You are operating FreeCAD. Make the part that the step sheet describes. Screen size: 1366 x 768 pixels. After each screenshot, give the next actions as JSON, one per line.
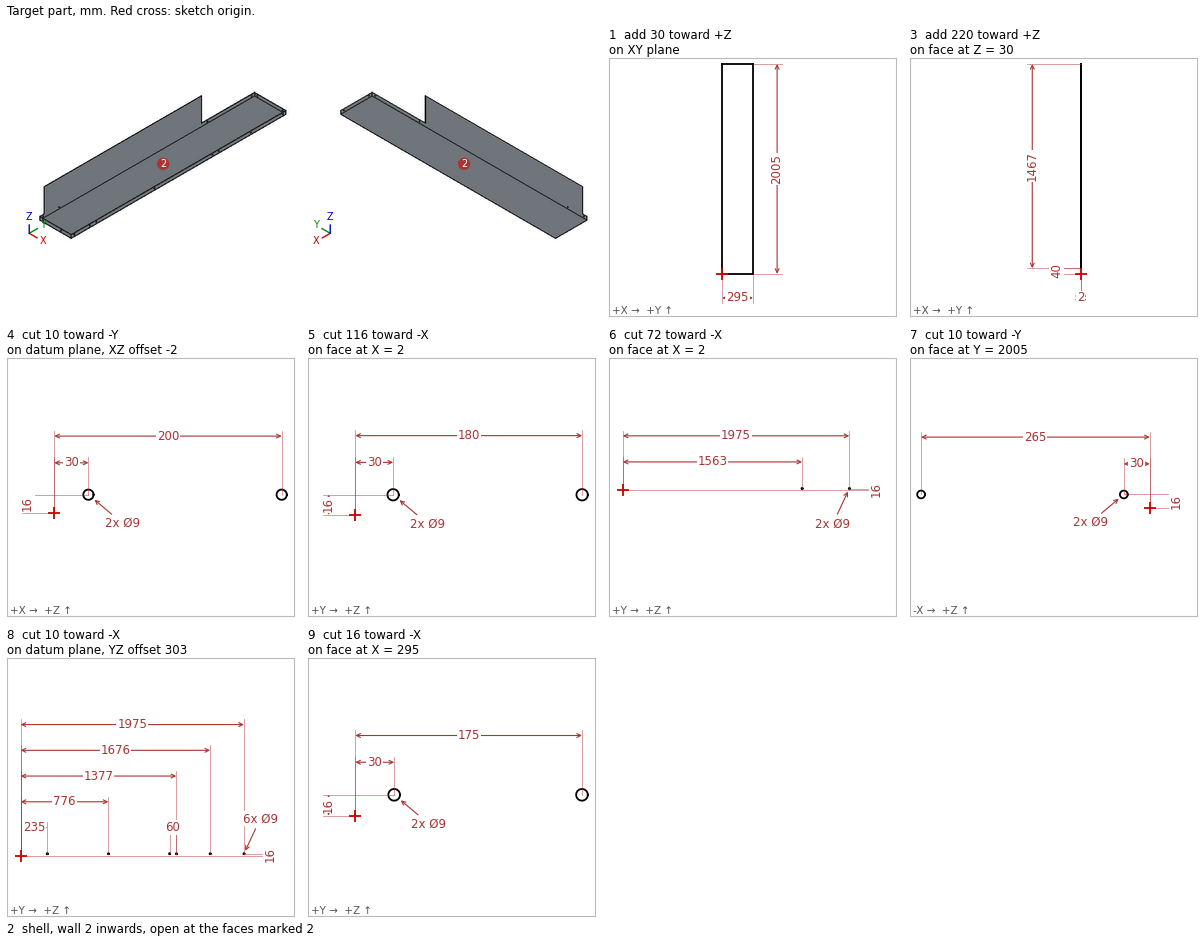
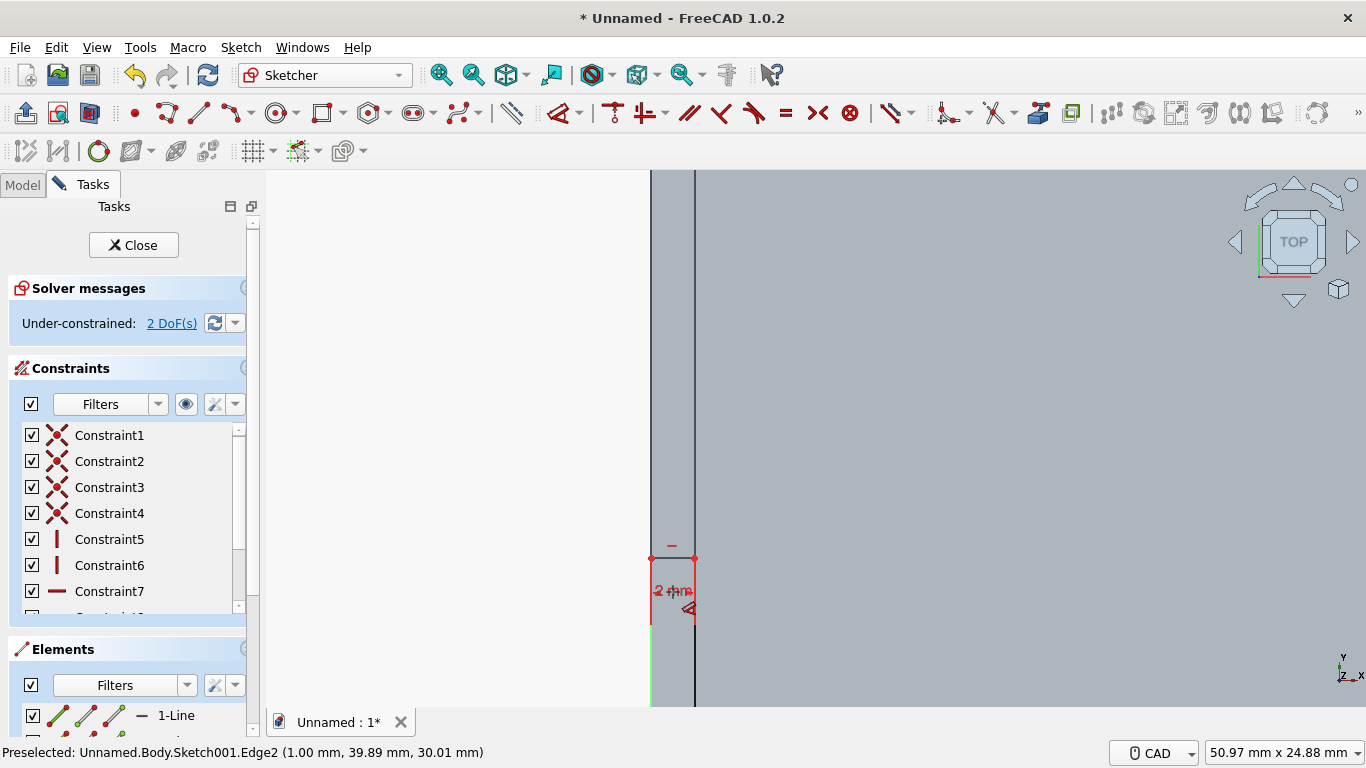
{"action": "scroll", "coordinate": [748, 438], "scroll_direction": "down", "scroll_amount": 15}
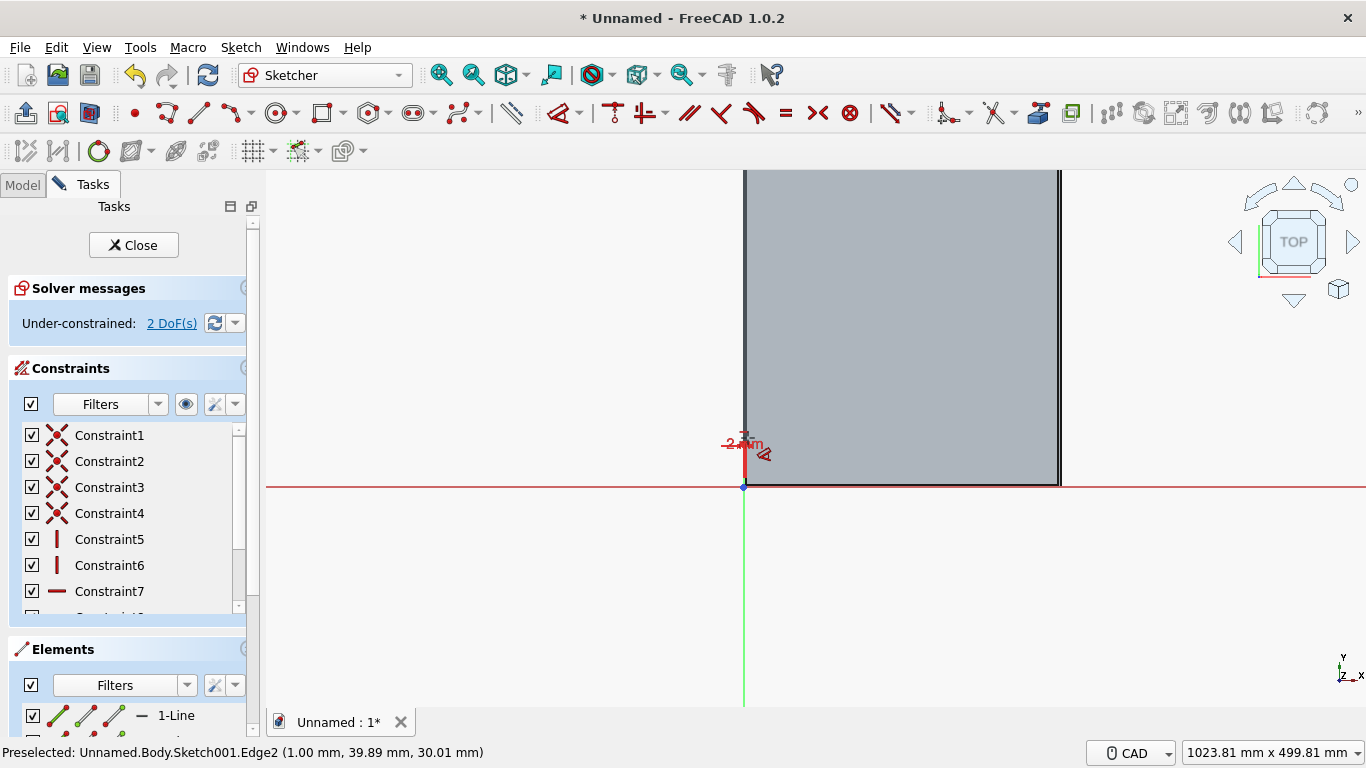
{"action": "scroll", "coordinate": [748, 631], "scroll_direction": "down", "scroll_amount": 8}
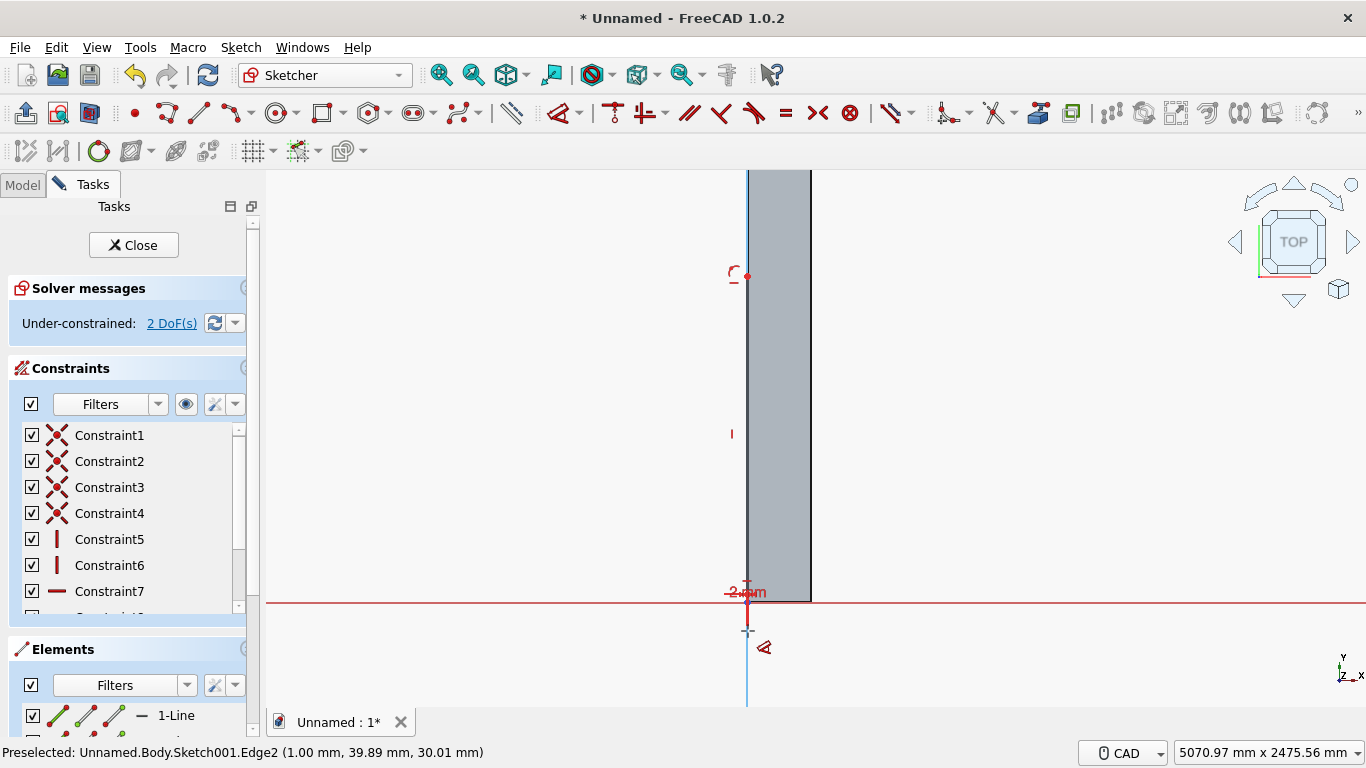
{"action": "scroll", "coordinate": [747, 594], "scroll_direction": "up", "scroll_amount": 14}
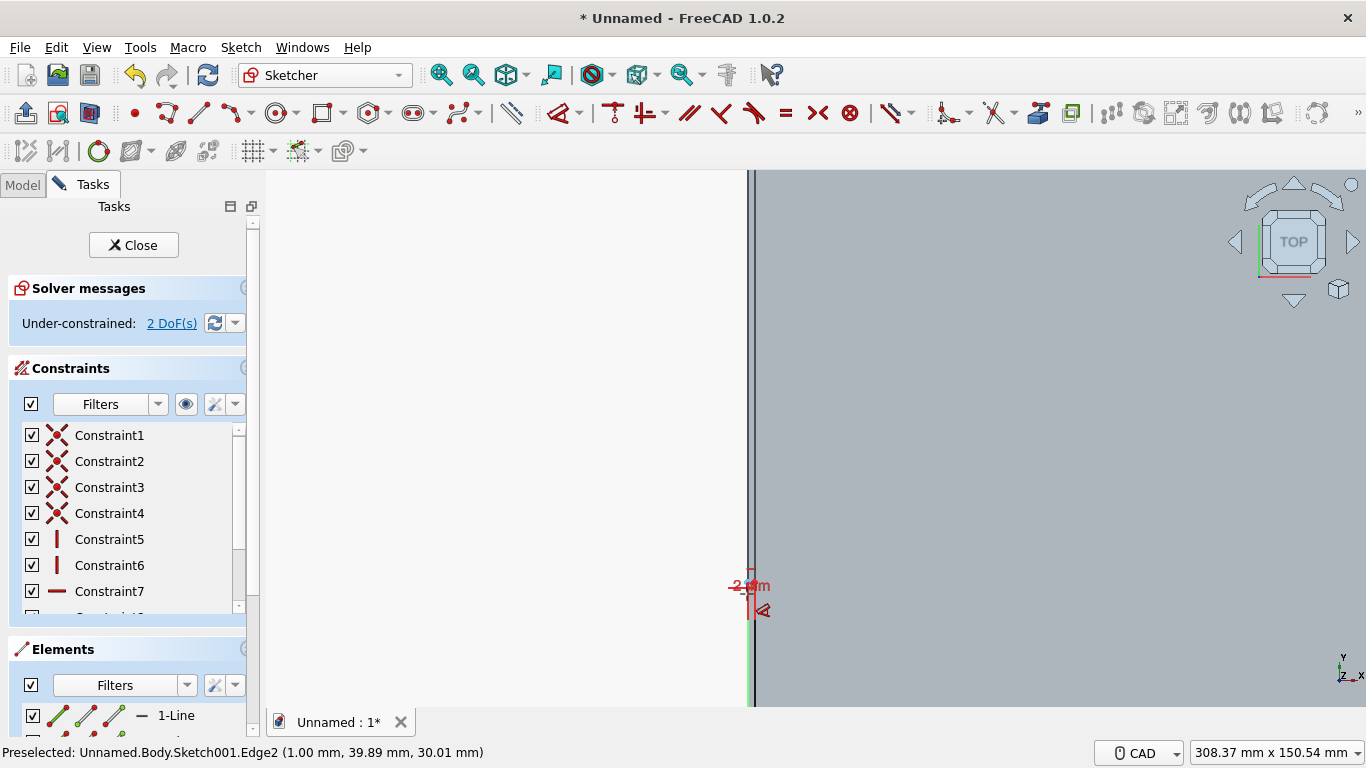
{"action": "left_click", "coordinate": [748, 582]}
{"action": "left_click", "coordinate": [714, 631]}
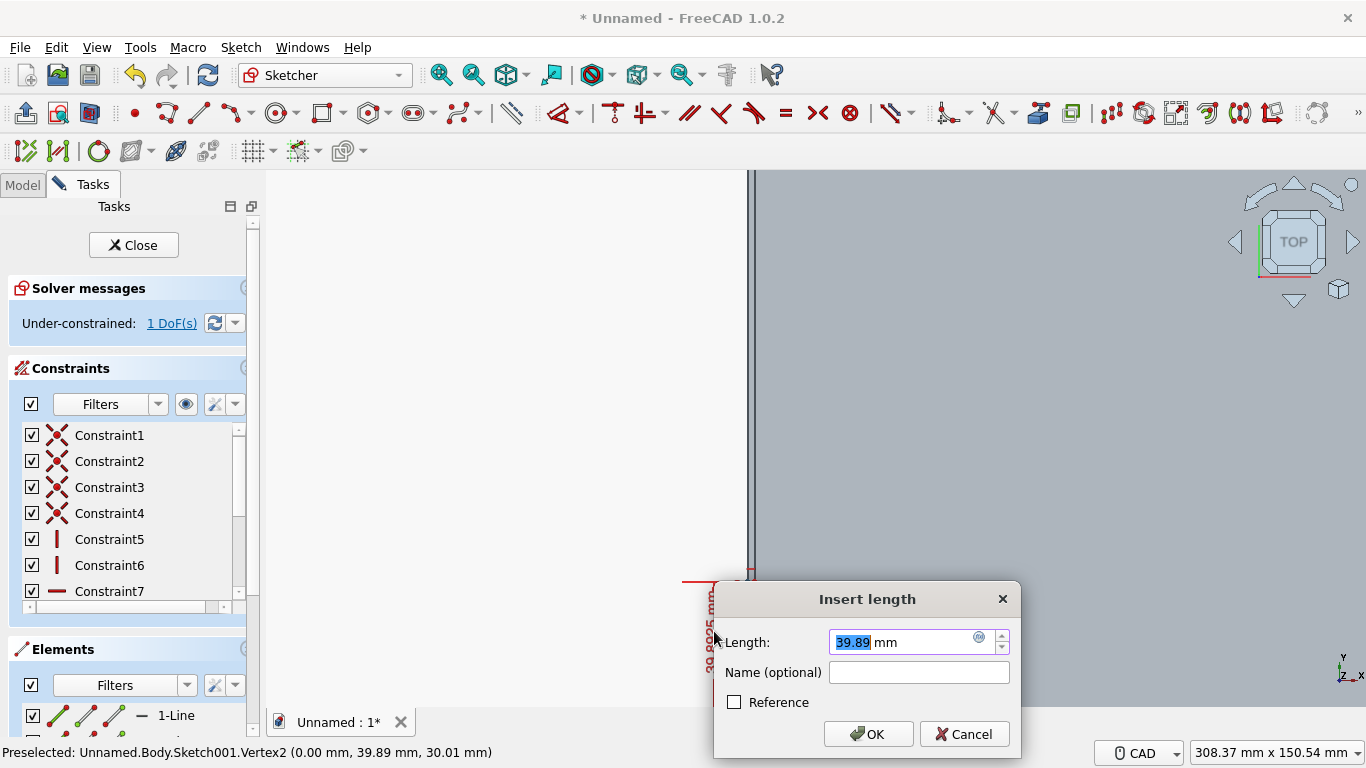
{"action": "type", "text": "40"}
{"action": "key", "text": "Return"}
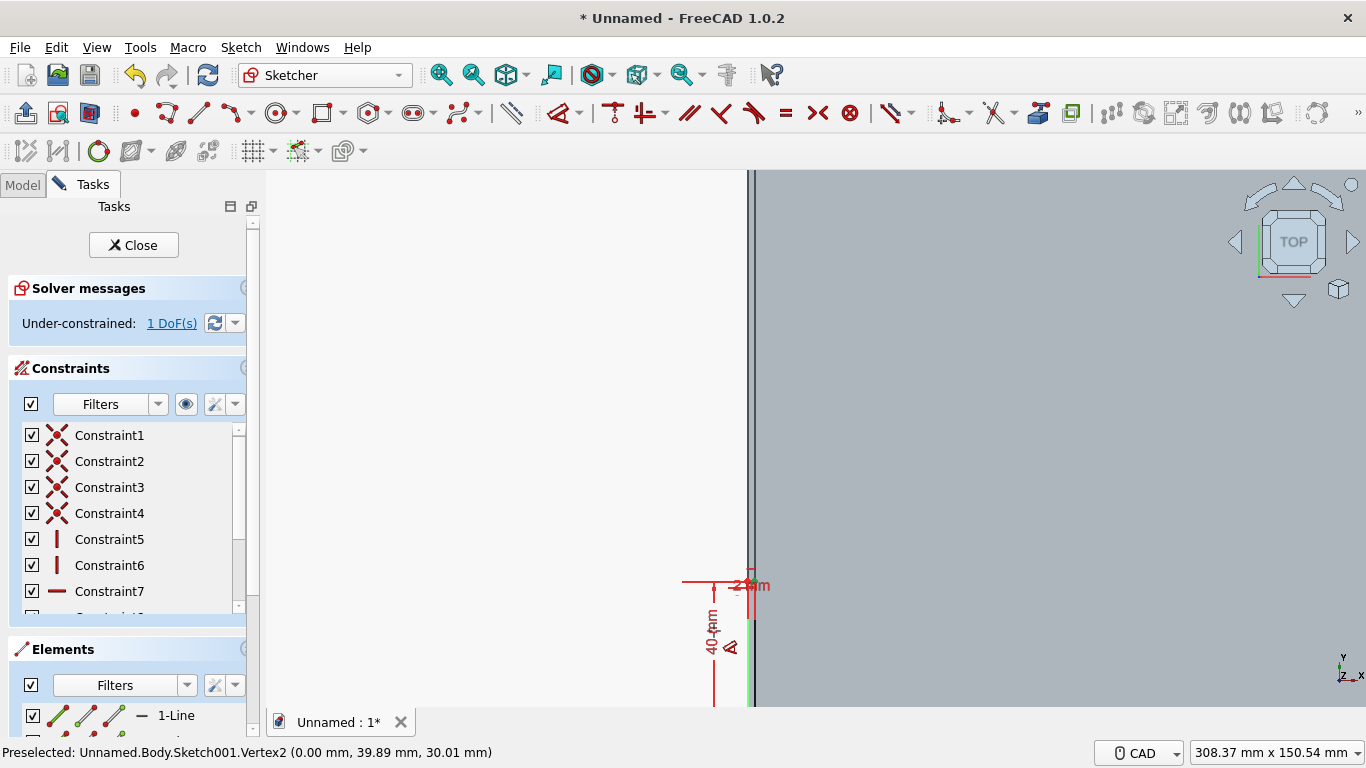
{"action": "scroll", "coordinate": [747, 594], "scroll_direction": "down", "scroll_amount": 14}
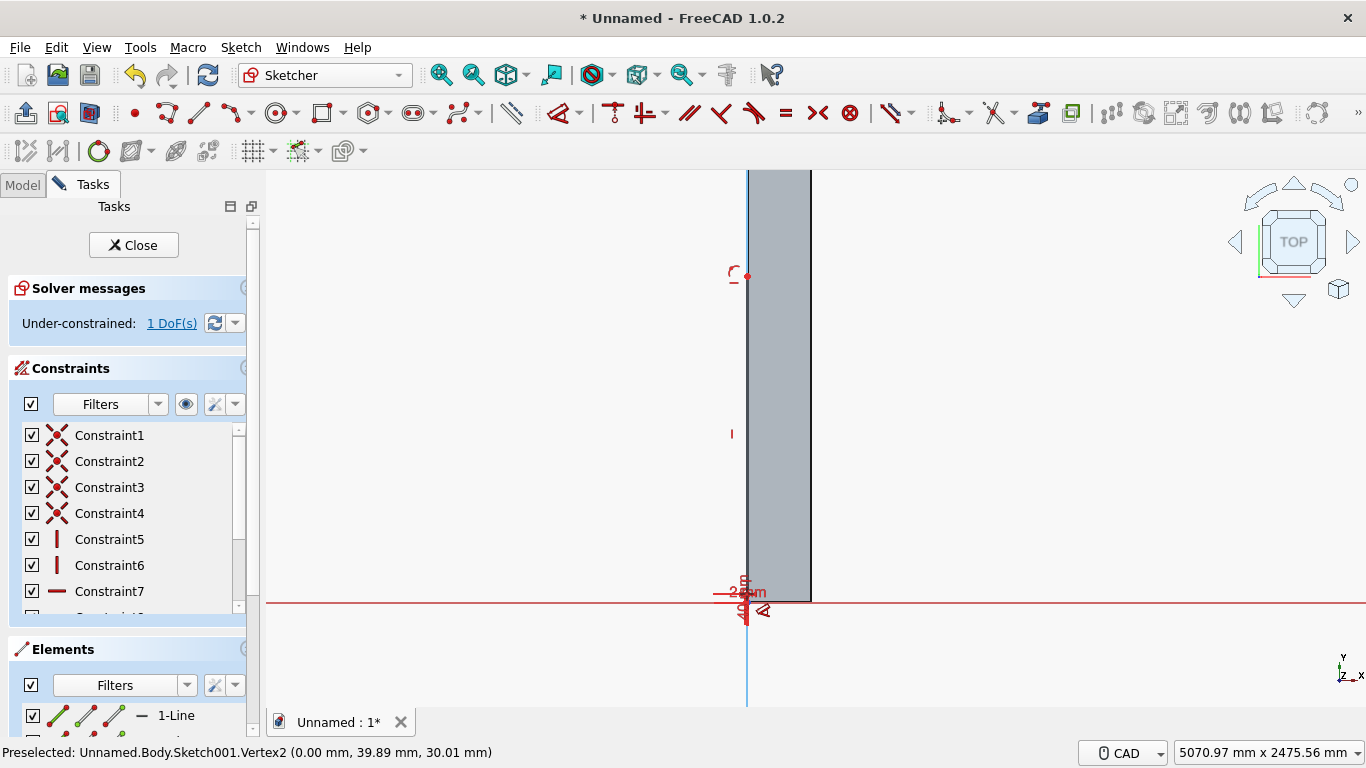
{"action": "scroll", "coordinate": [747, 372], "scroll_direction": "up", "scroll_amount": 14}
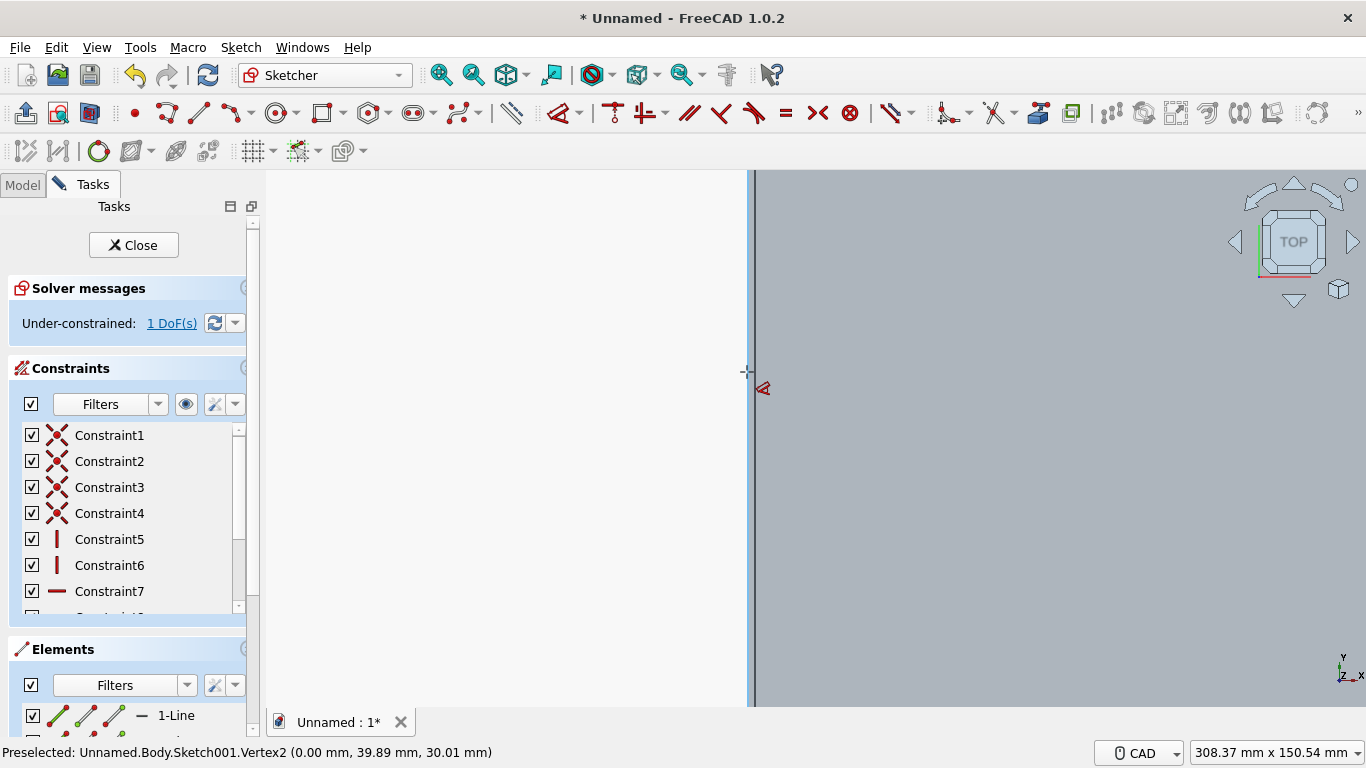
{"action": "left_click", "coordinate": [748, 361]}
{"action": "left_click", "coordinate": [714, 438]}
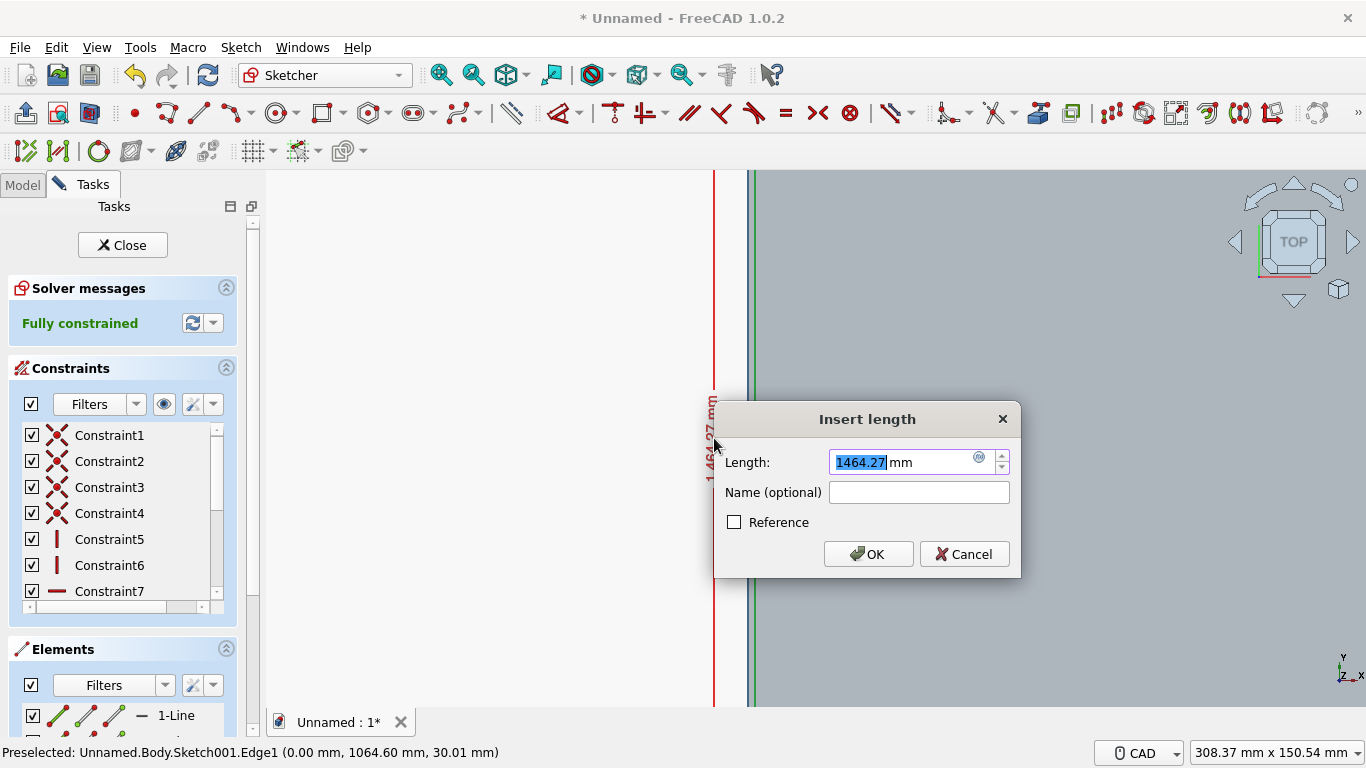
{"action": "type", "text": "1467"}
{"action": "key", "text": "Return"}
{"action": "key", "text": "Escape"}